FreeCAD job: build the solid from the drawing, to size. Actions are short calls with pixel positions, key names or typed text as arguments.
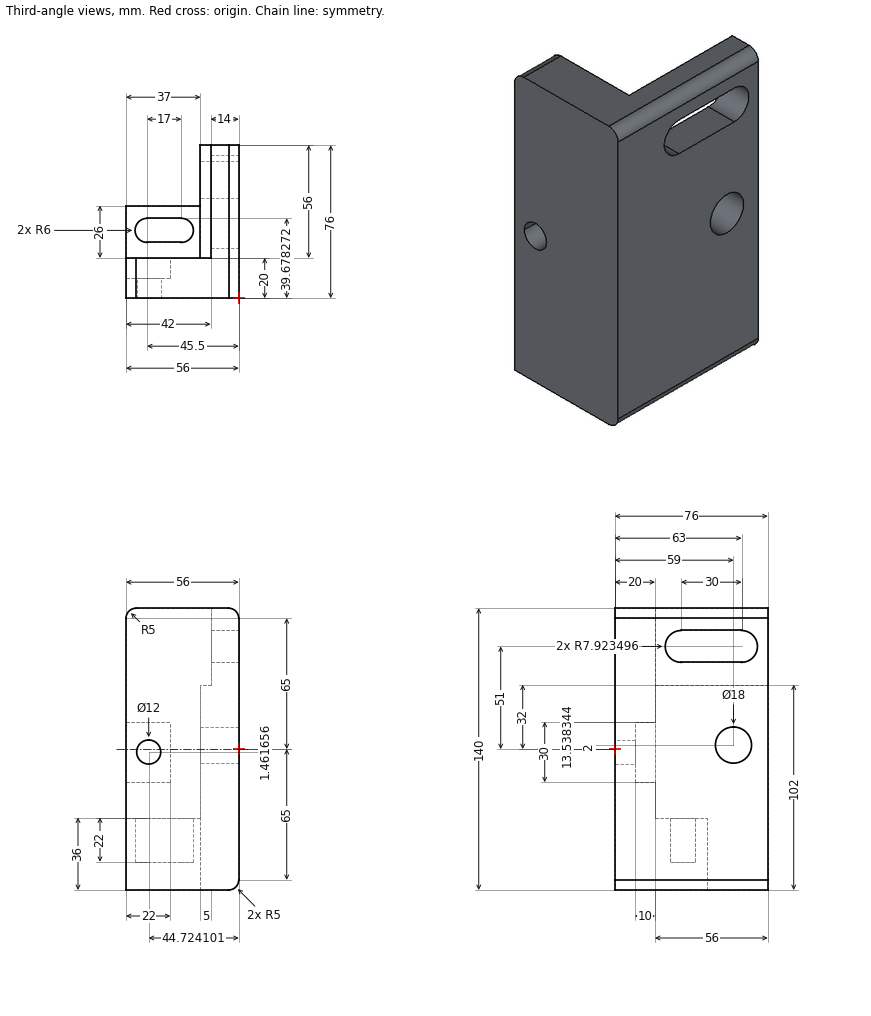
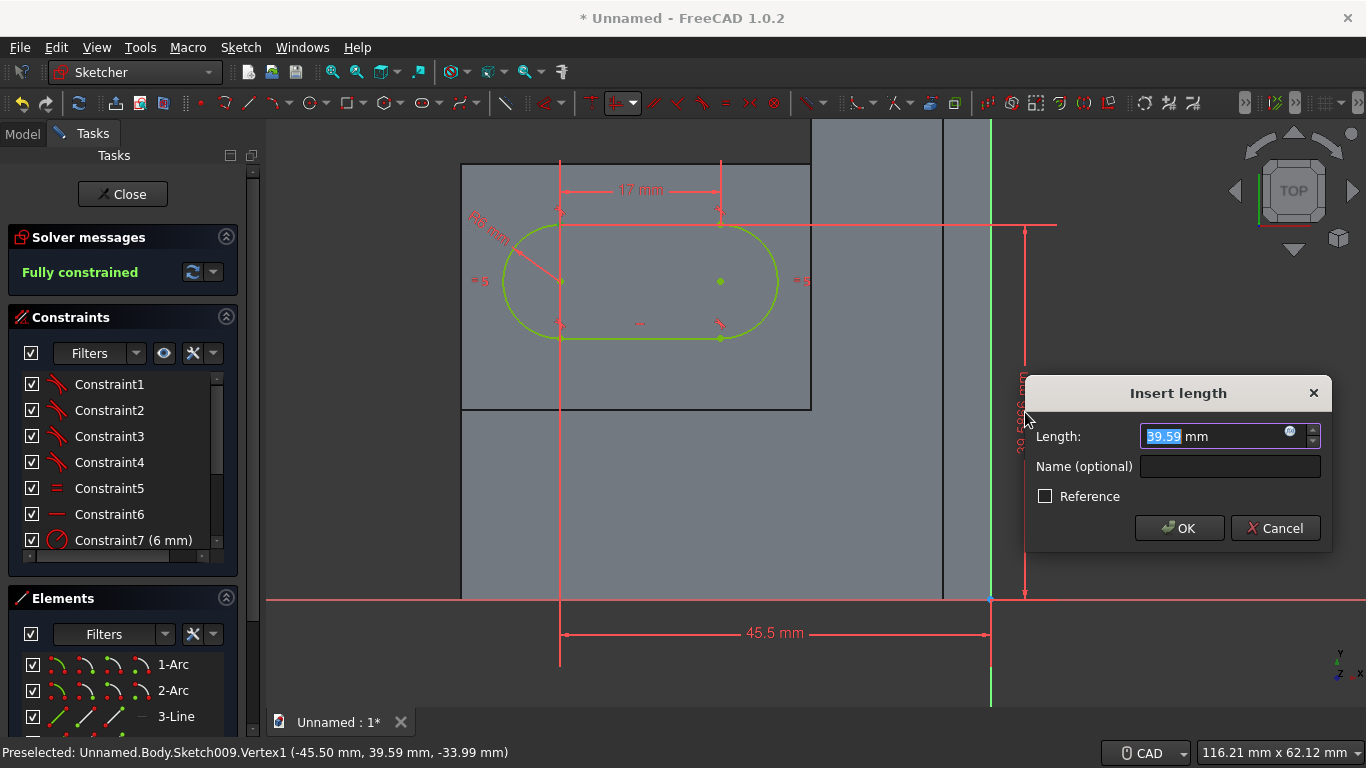
text(39.678272)
key(Return)
key(Escape)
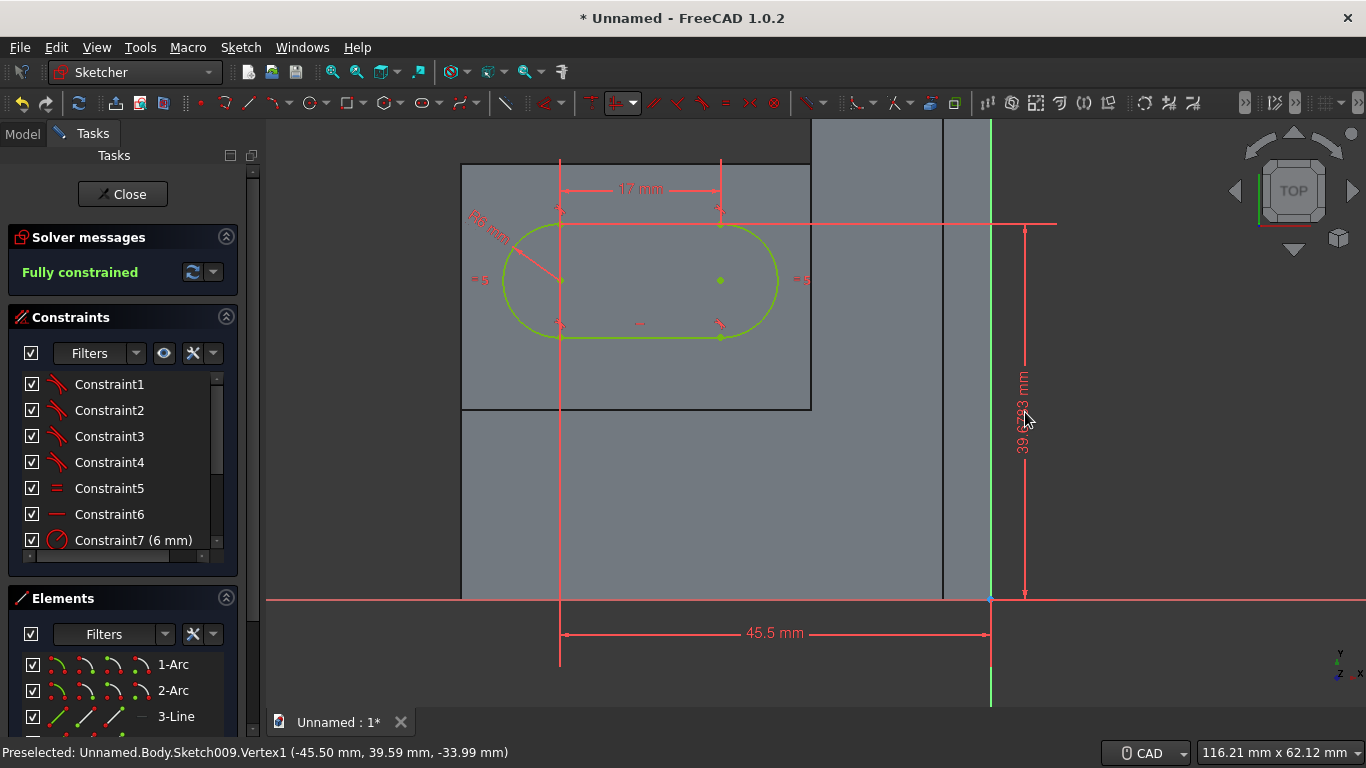
click(123, 194)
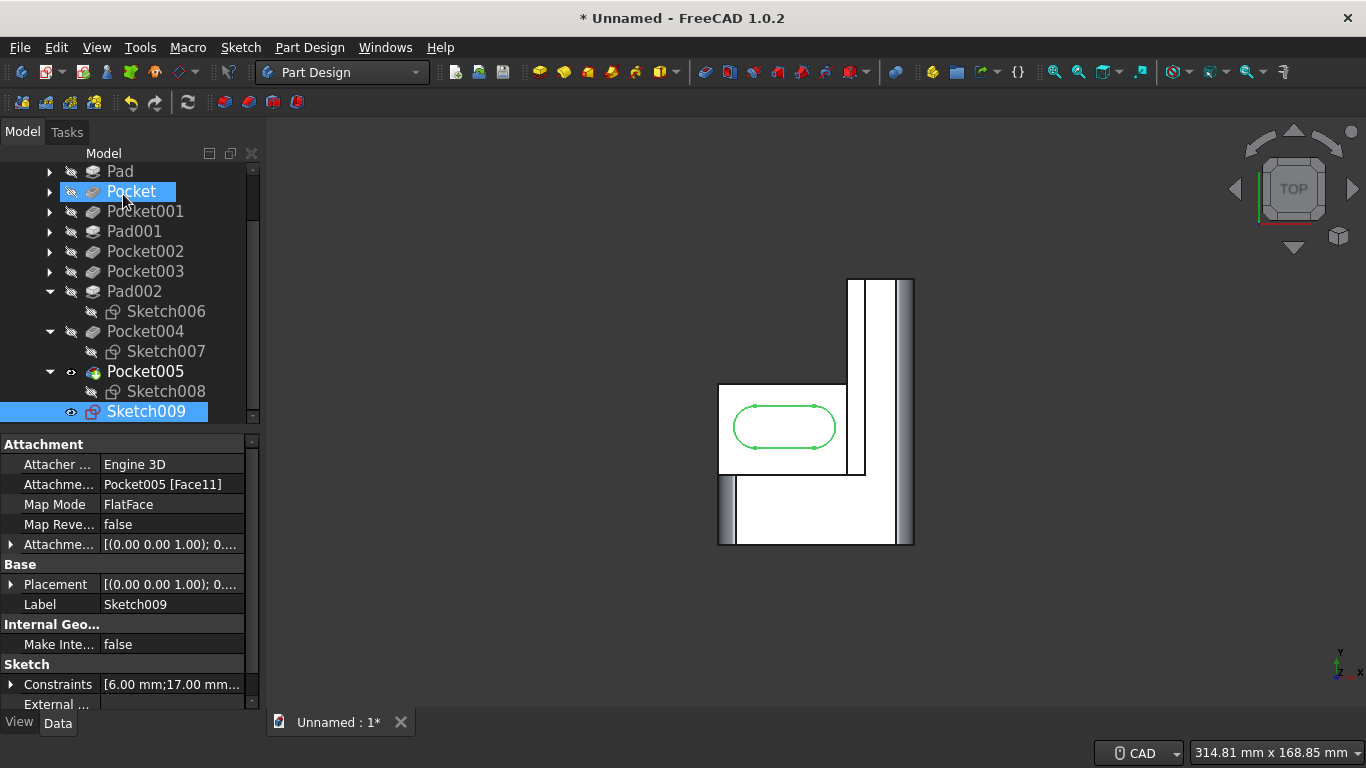
click(706, 72)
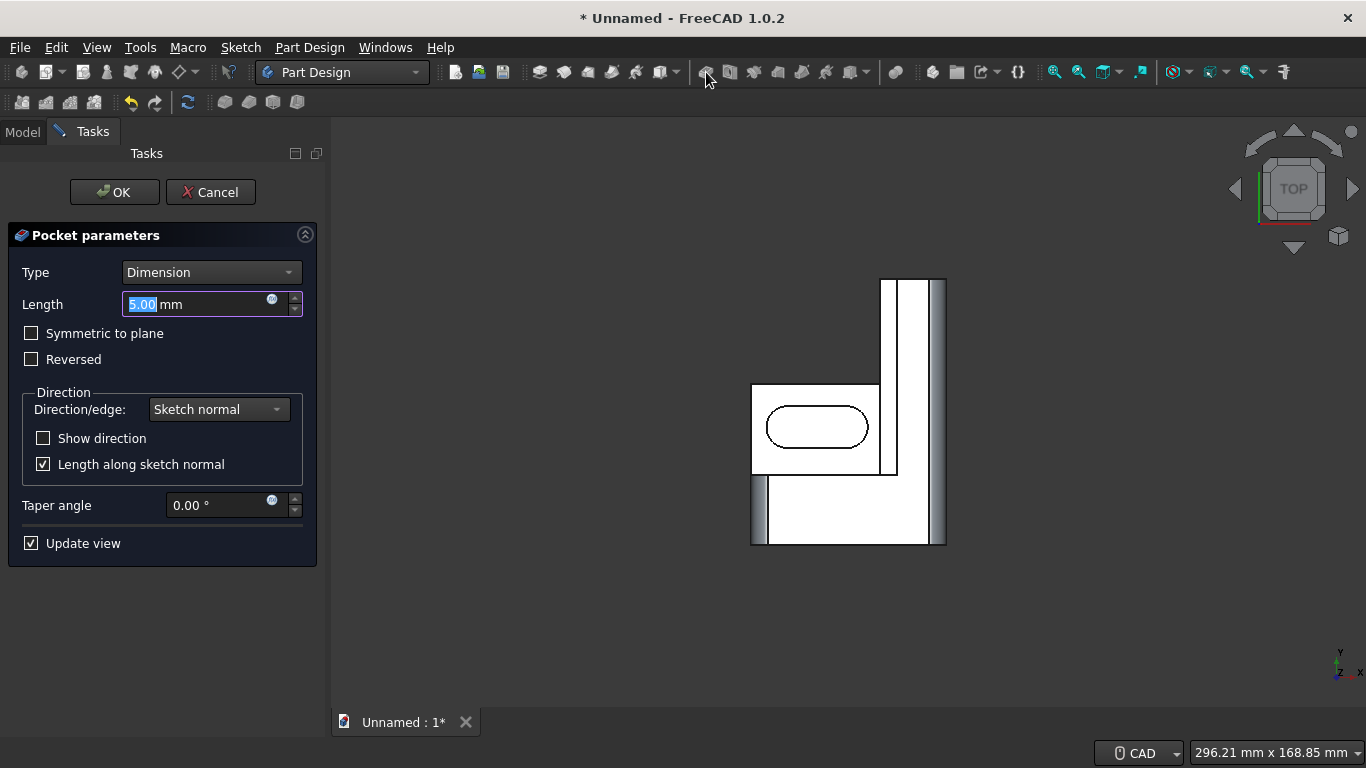
text(22)
key(Tab)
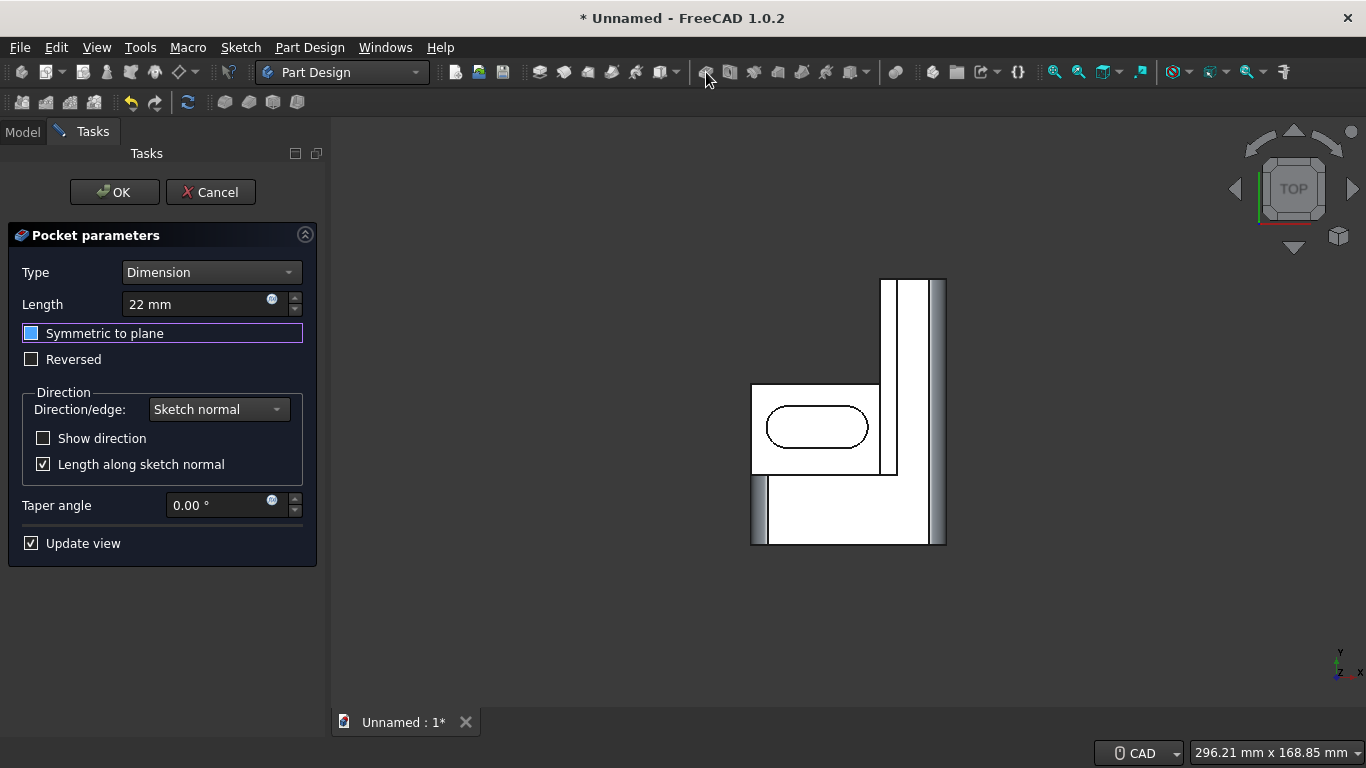
click(115, 192)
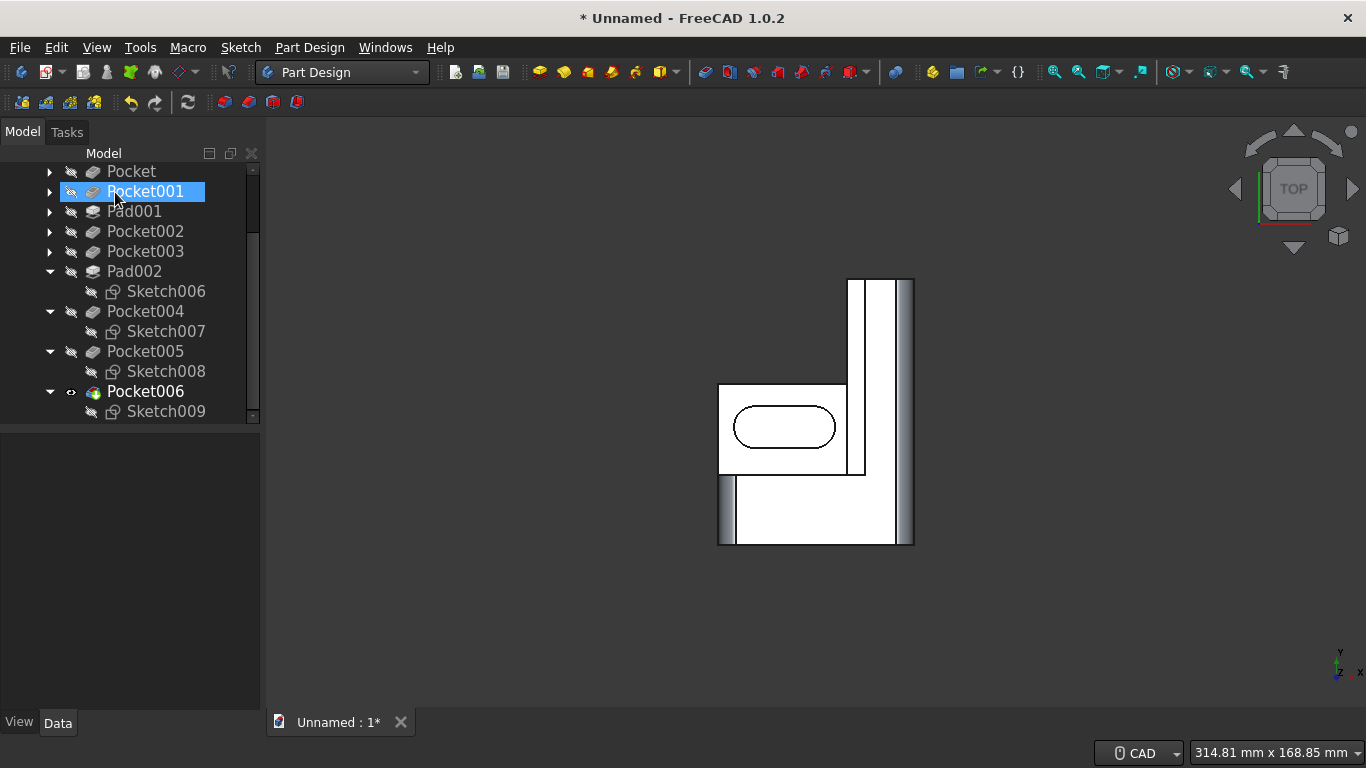
key(0)